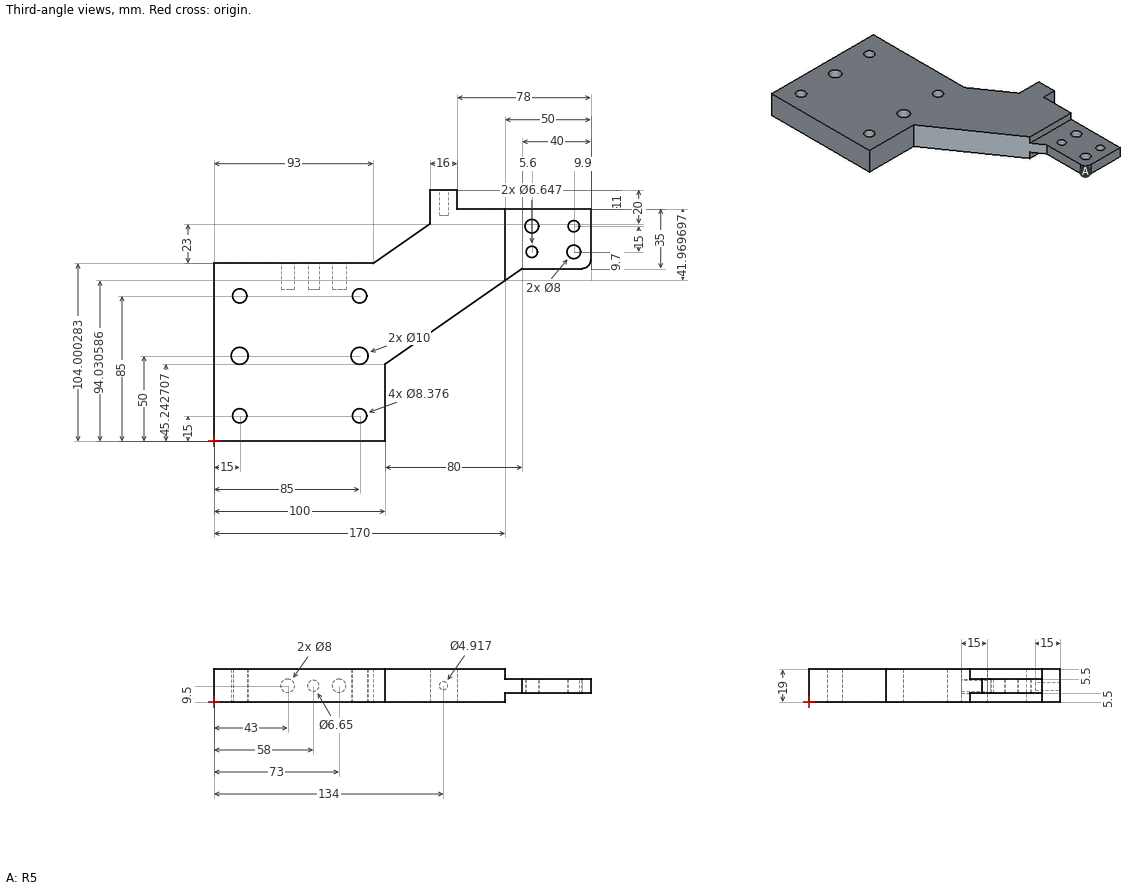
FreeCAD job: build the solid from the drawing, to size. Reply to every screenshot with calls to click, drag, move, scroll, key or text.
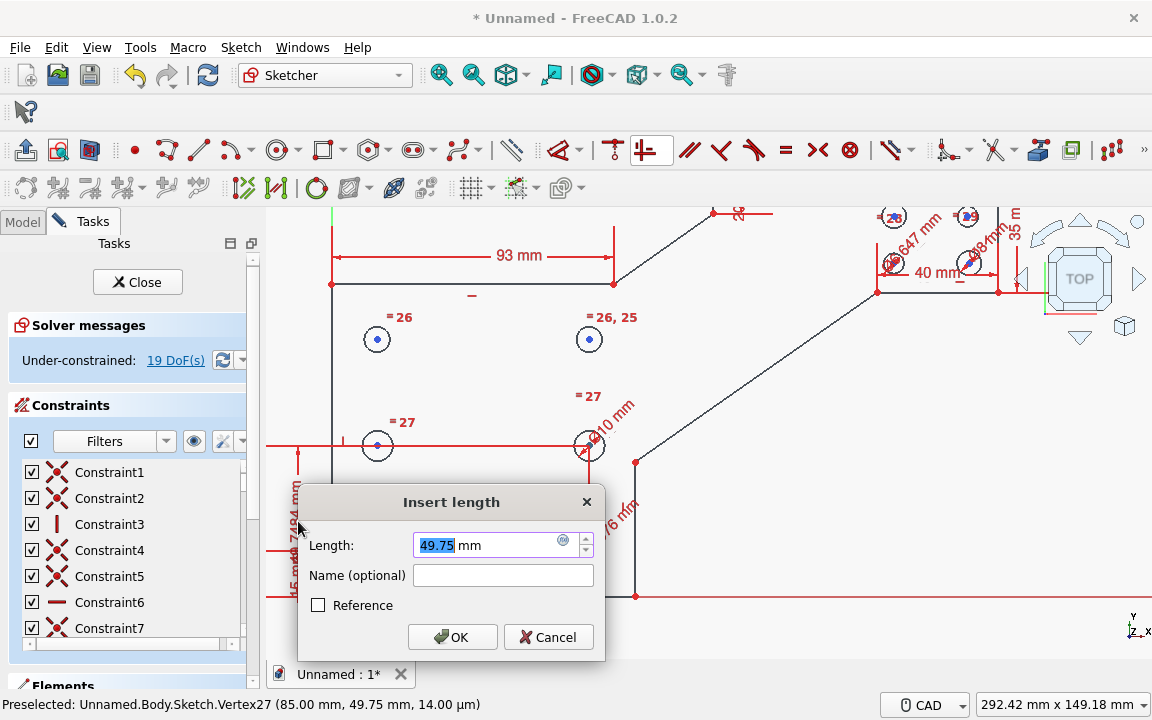
text(50)
key(Return)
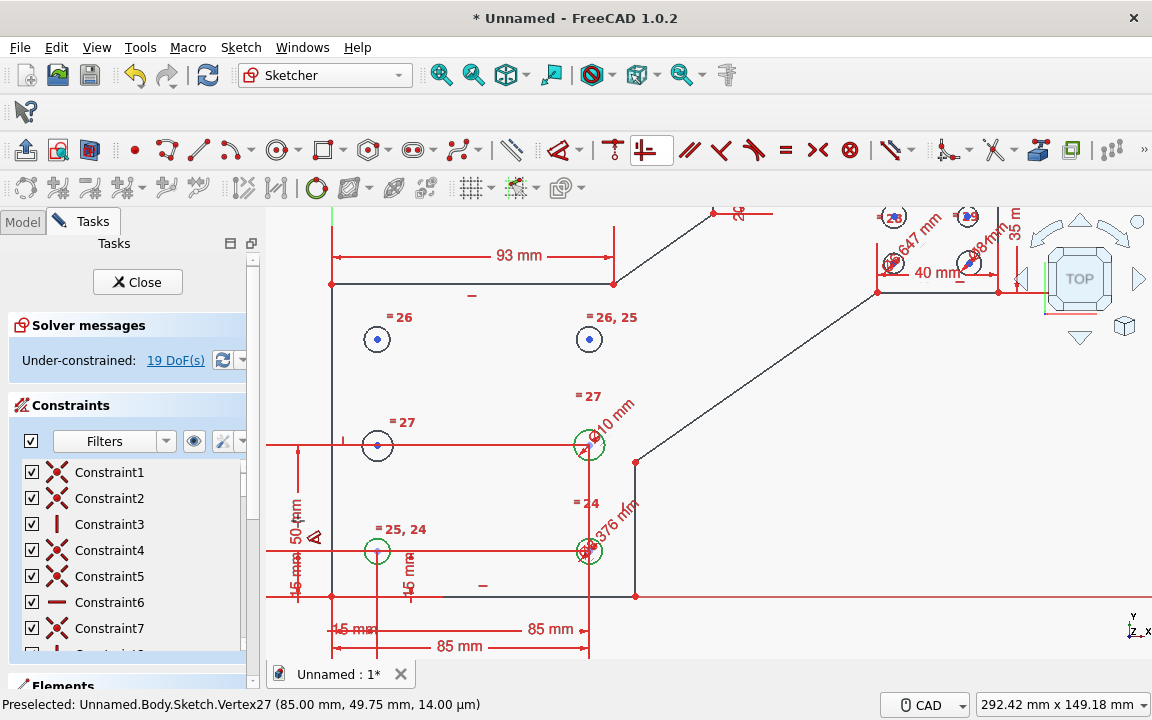
click(378, 446)
click(355, 412)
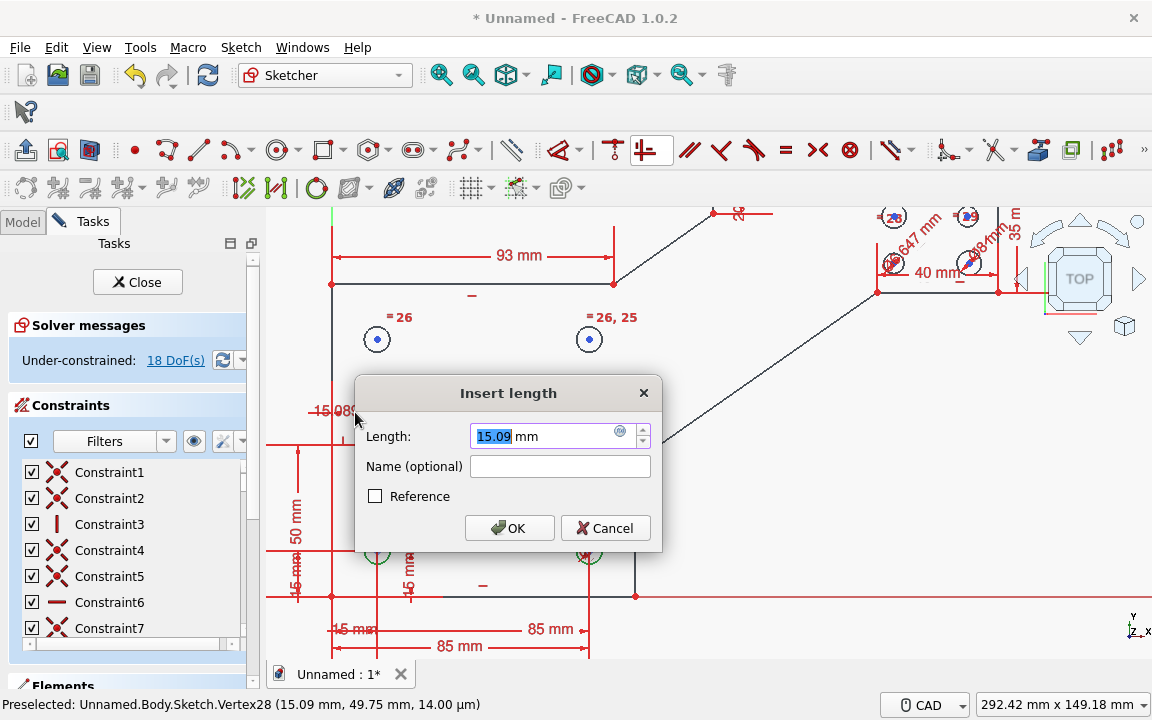
text(15)
key(Return)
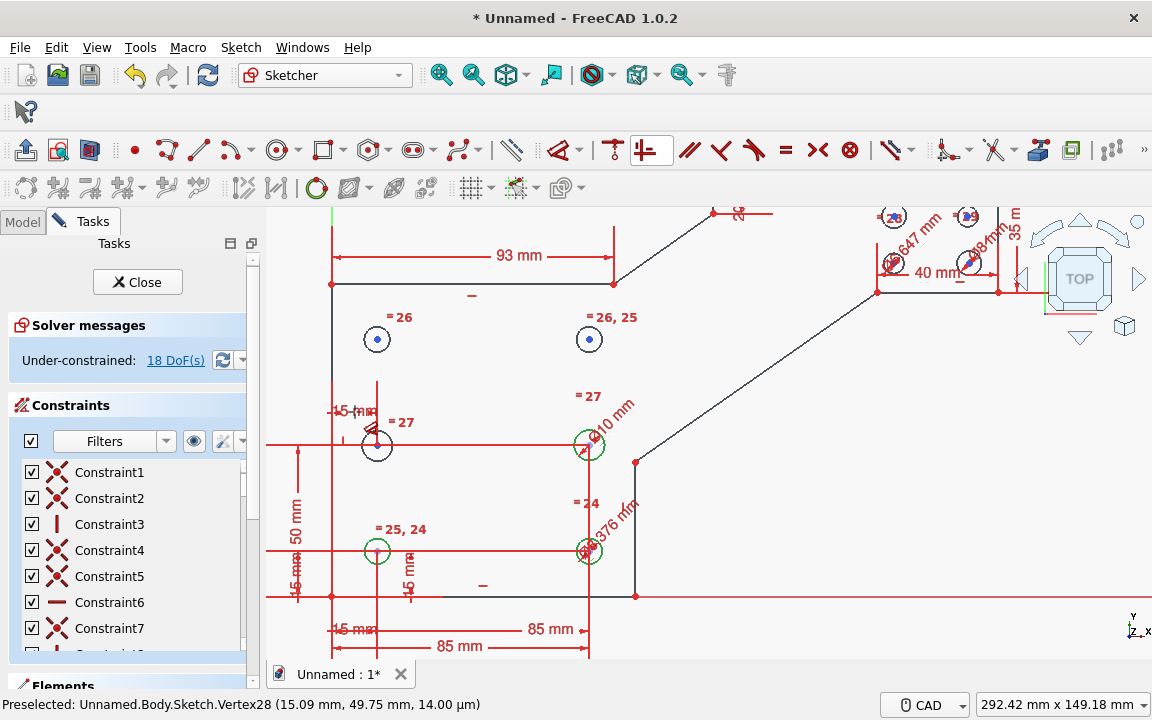
click(377, 446)
click(298, 487)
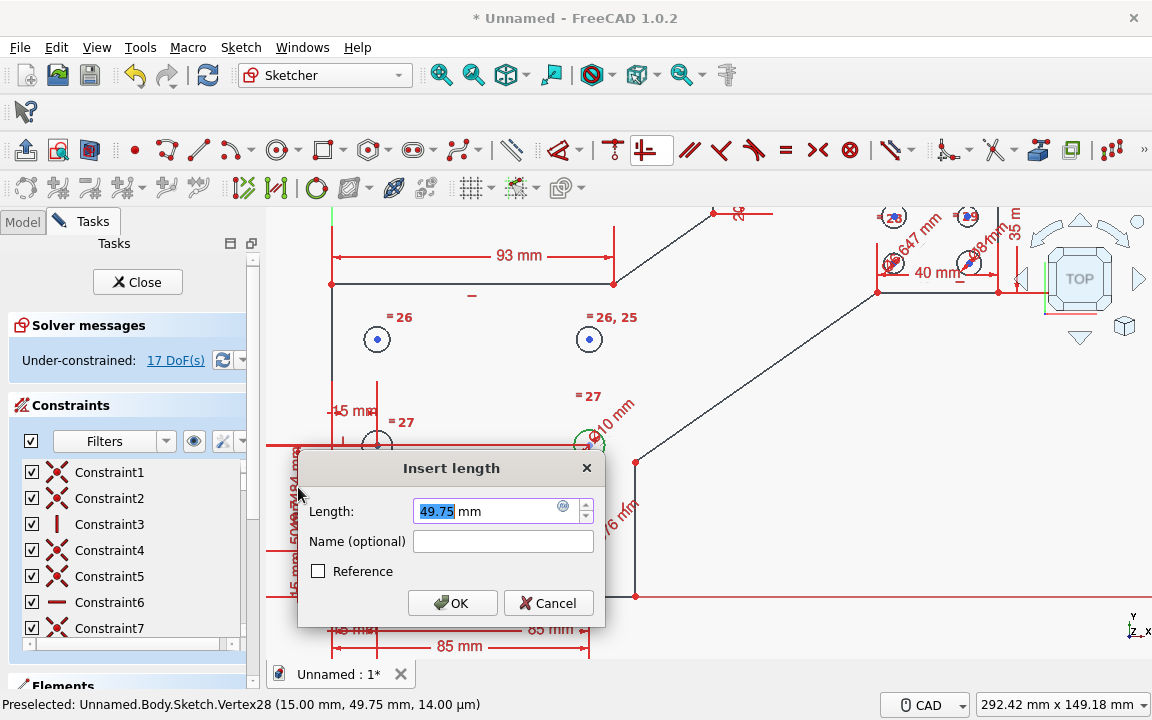
text(50)
key(Return)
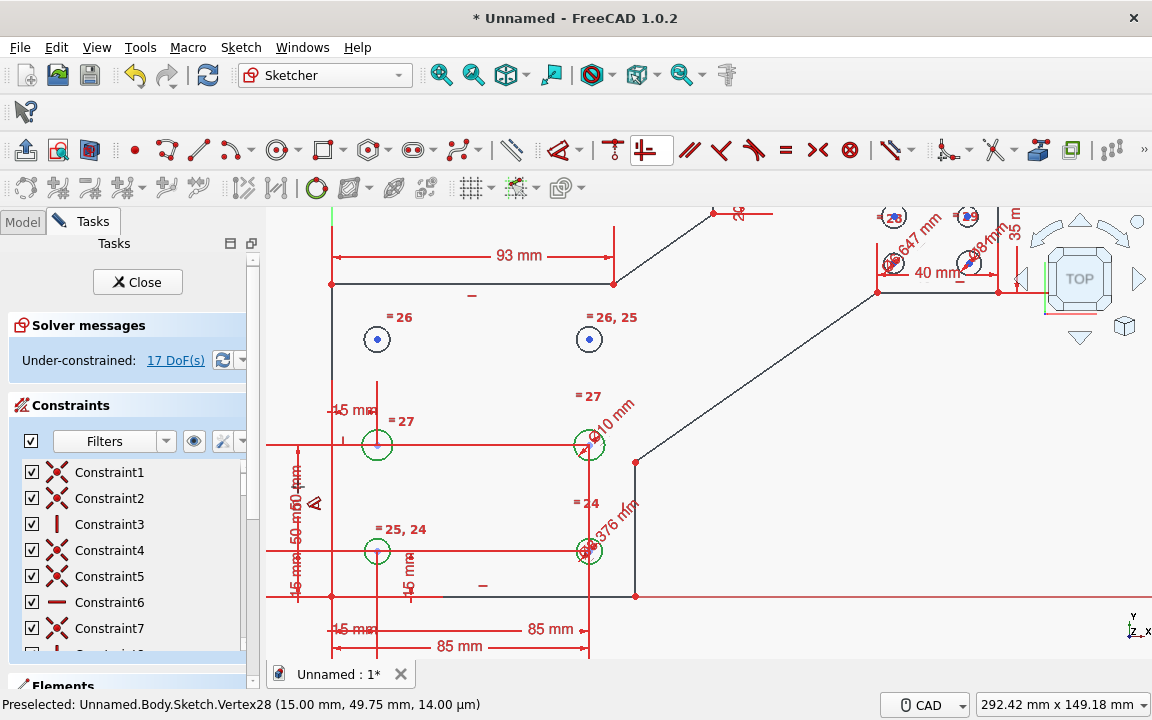
click(589, 340)
click(461, 306)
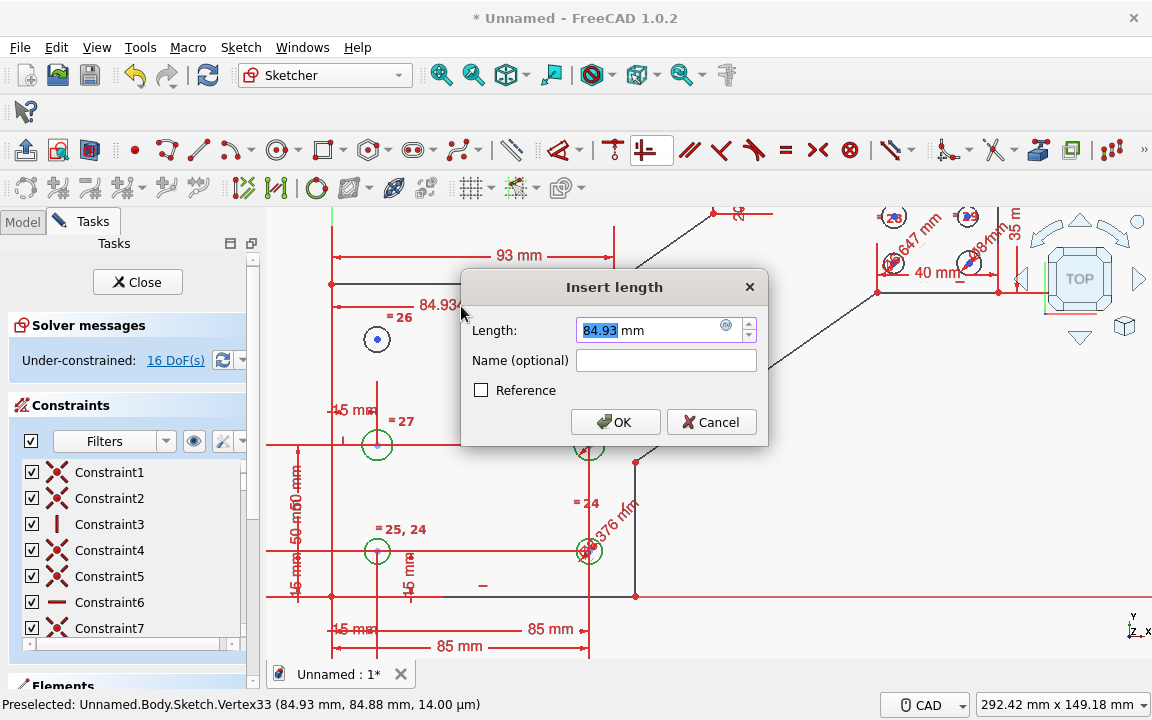
text(85)
key(Return)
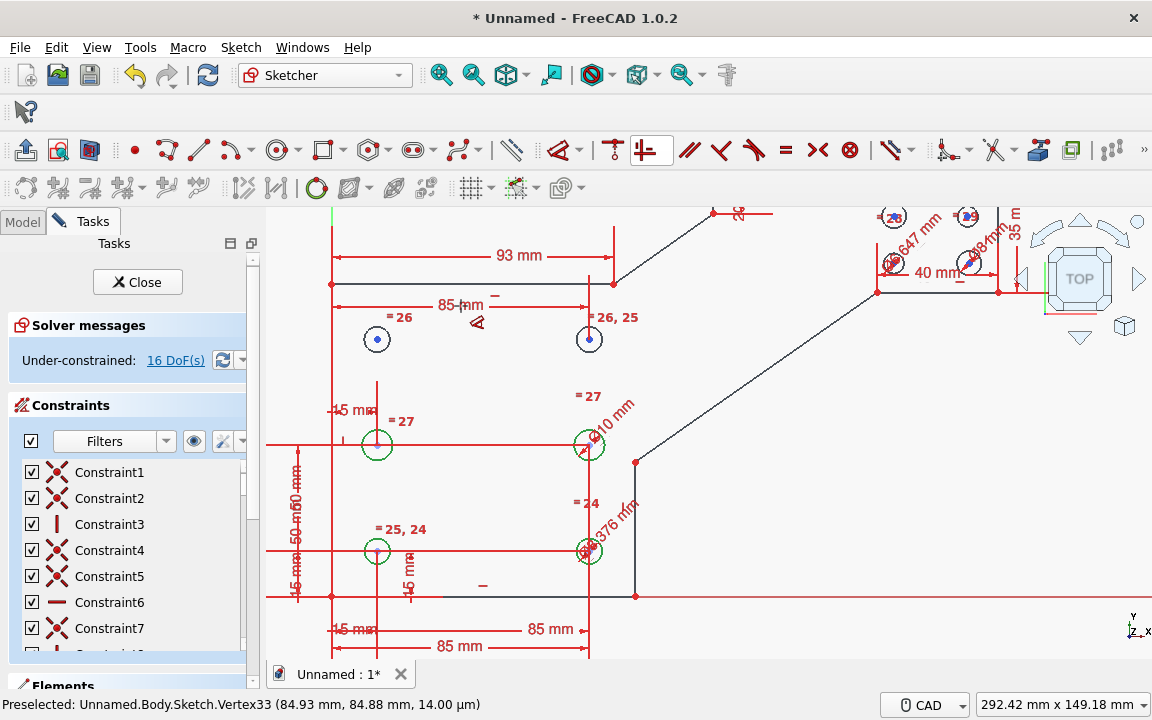
click(589, 340)
click(298, 378)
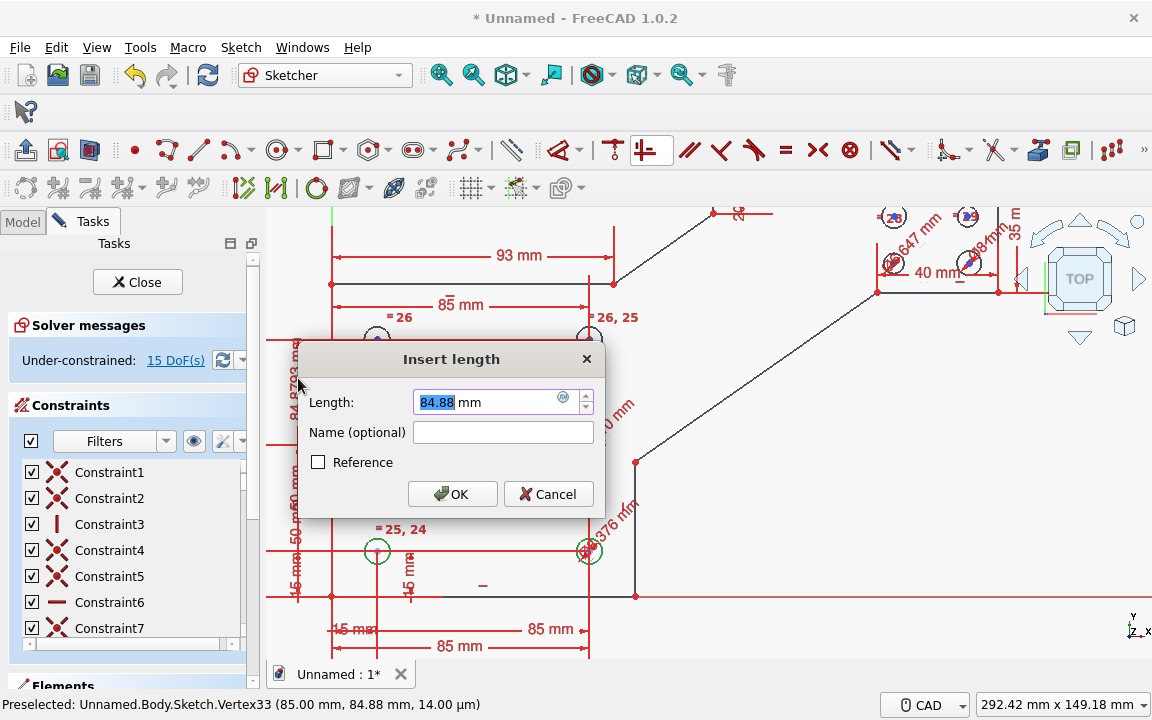
text(85)
key(Return)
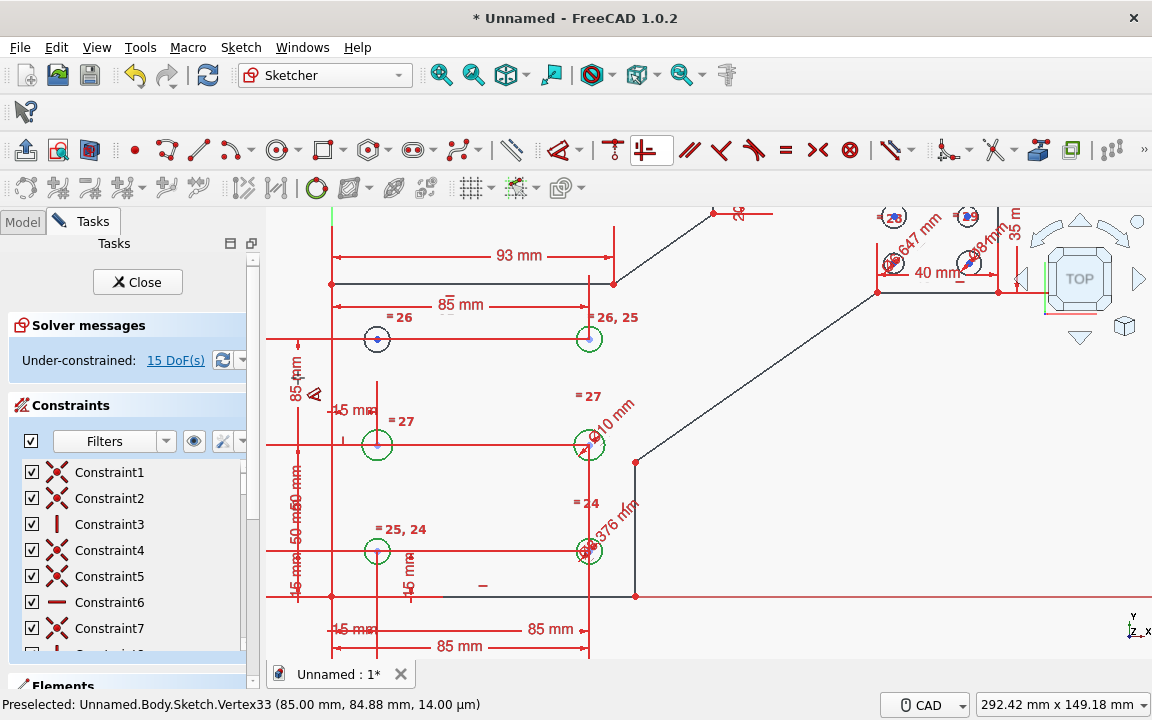
click(377, 340)
click(354, 306)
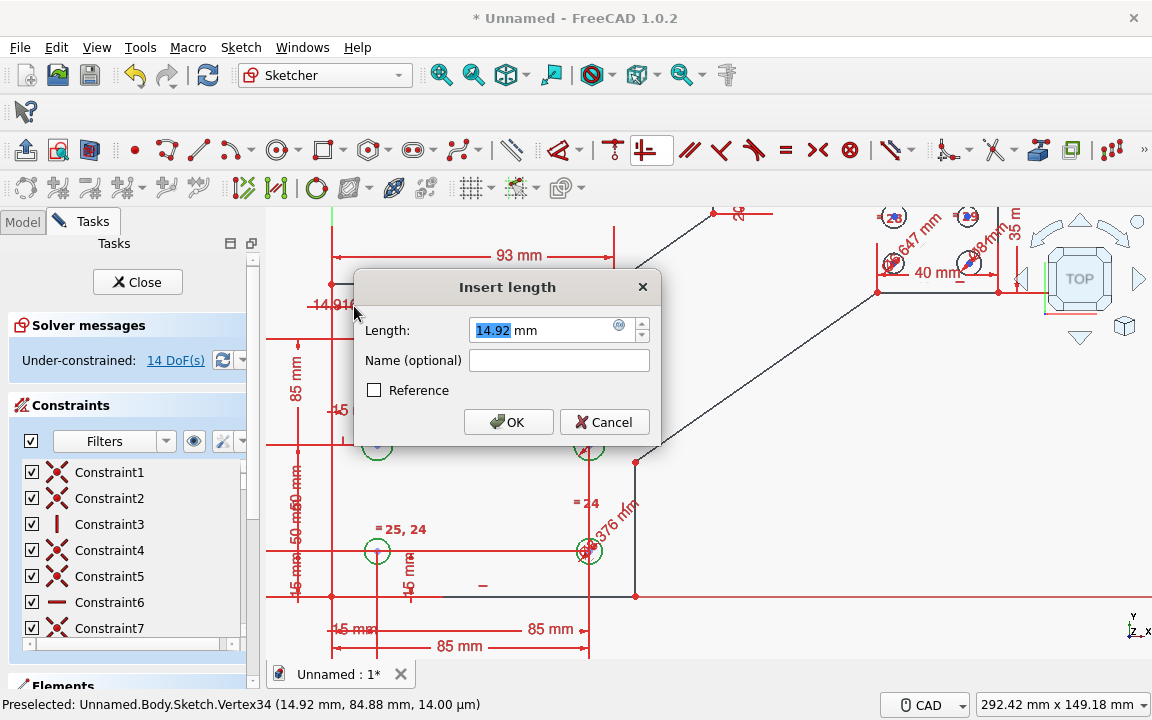
text(15)
key(Return)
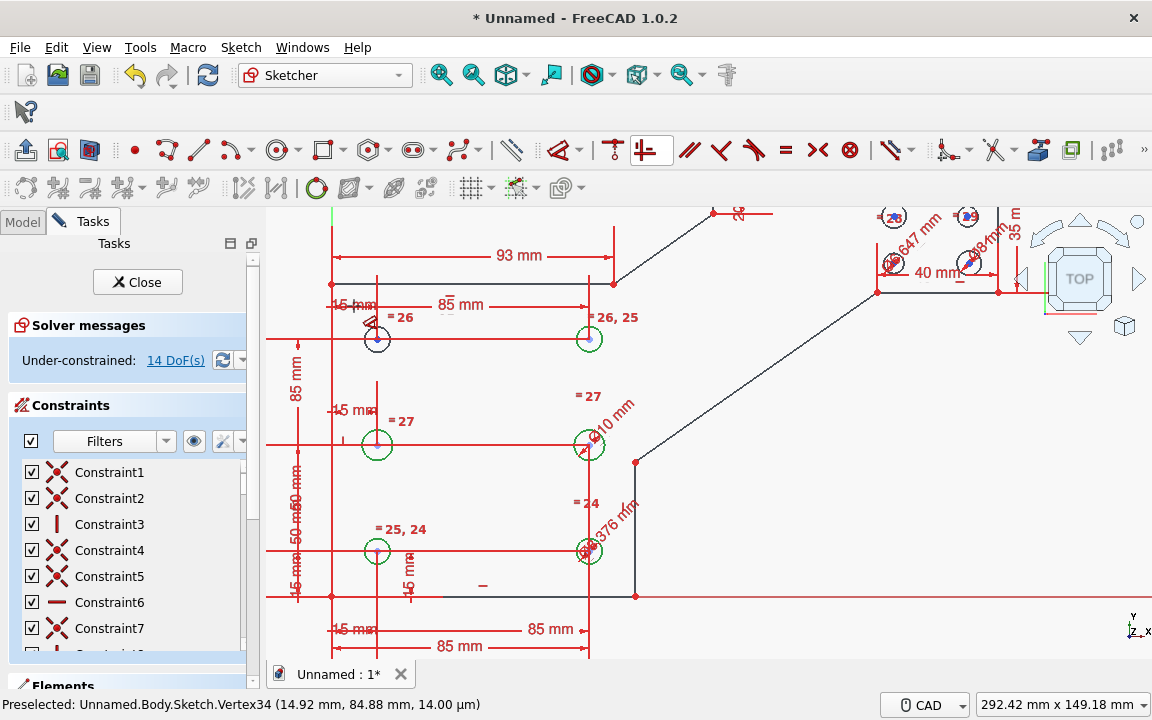
click(377, 340)
click(411, 468)